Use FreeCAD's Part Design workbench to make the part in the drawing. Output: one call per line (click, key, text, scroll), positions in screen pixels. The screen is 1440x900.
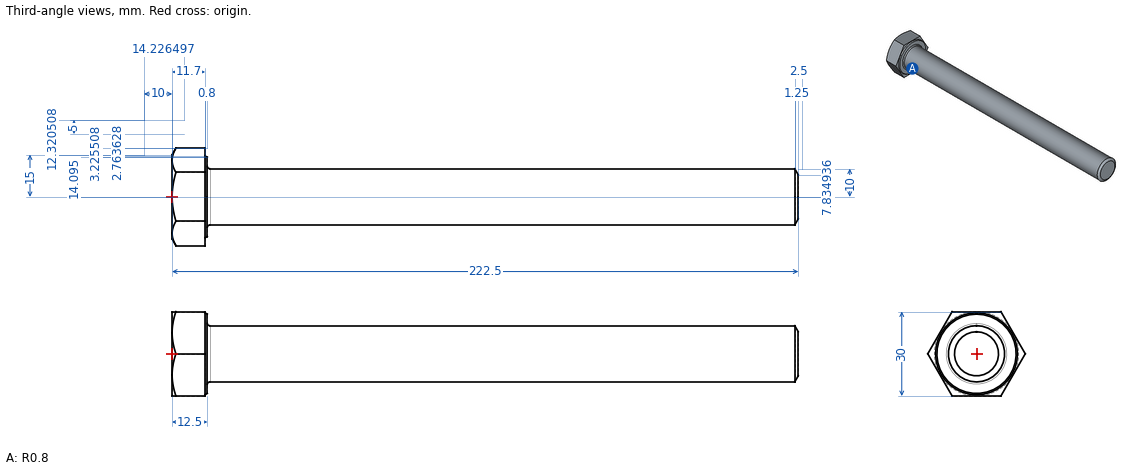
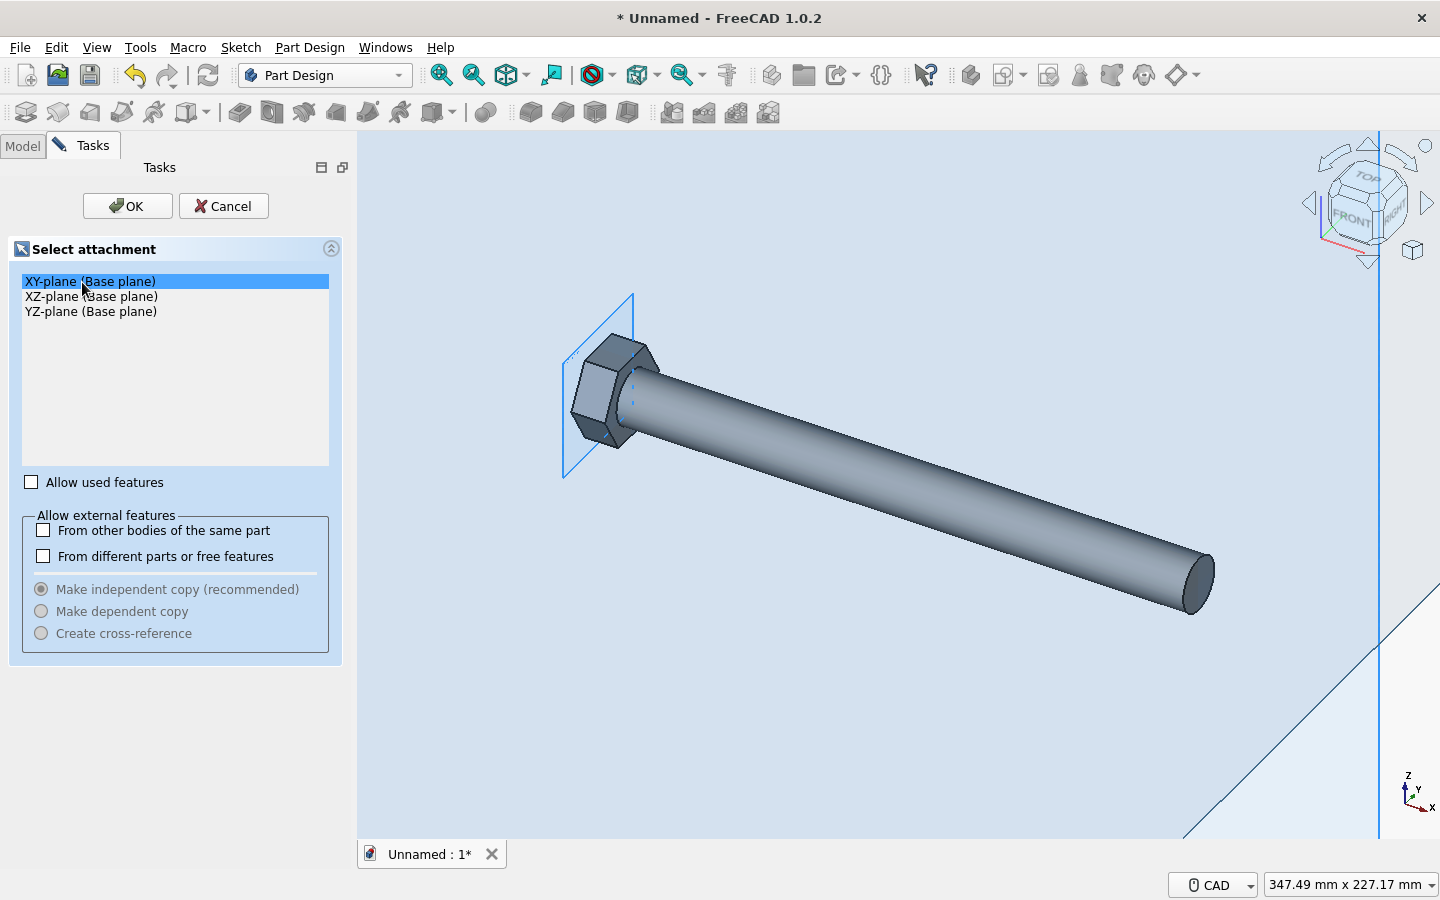
click(128, 206)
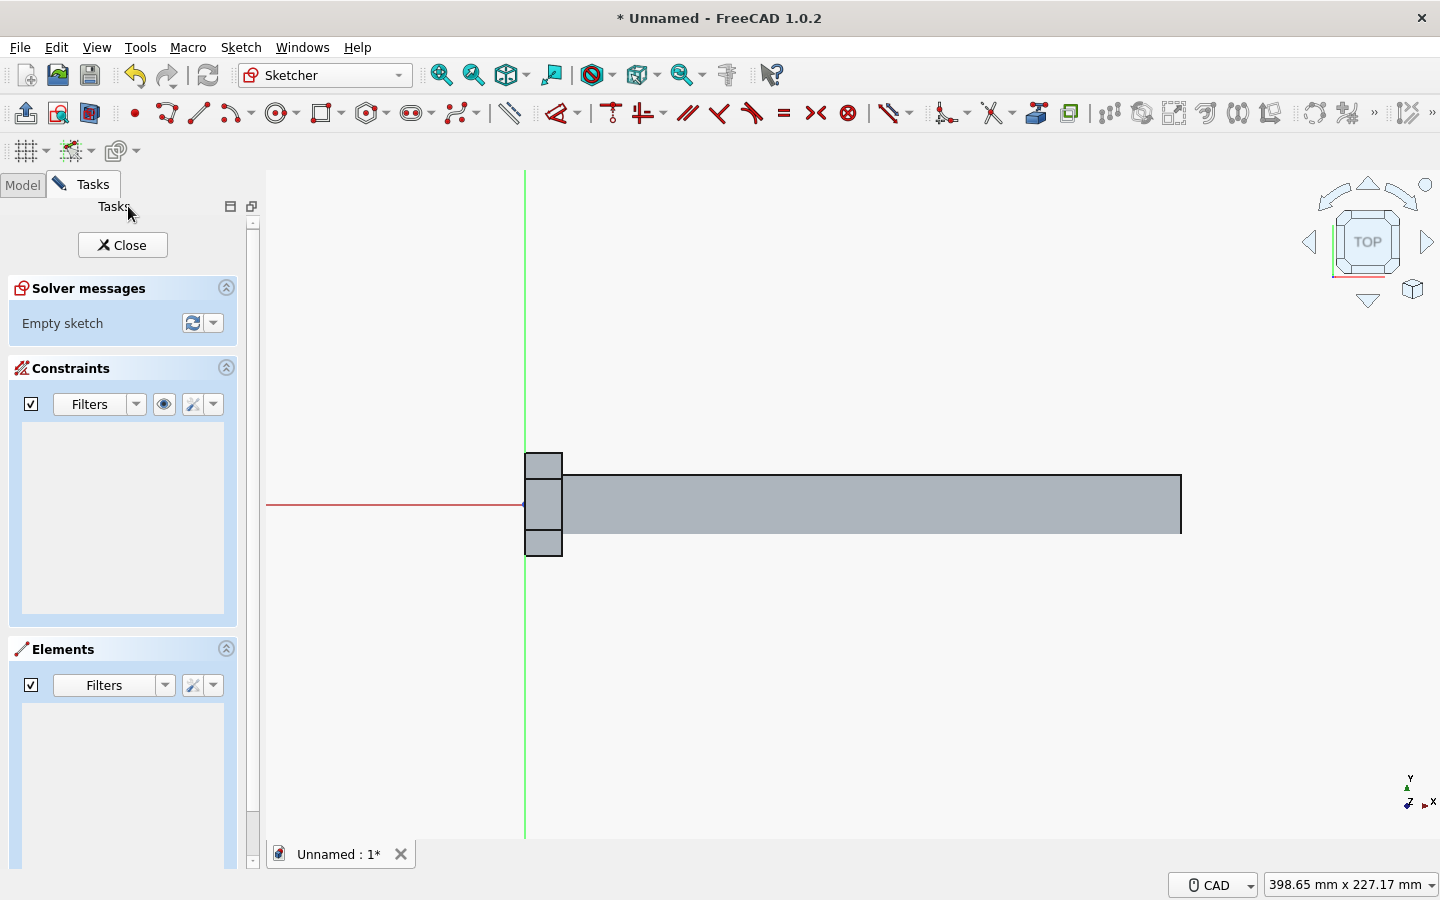
key(q)
key(s)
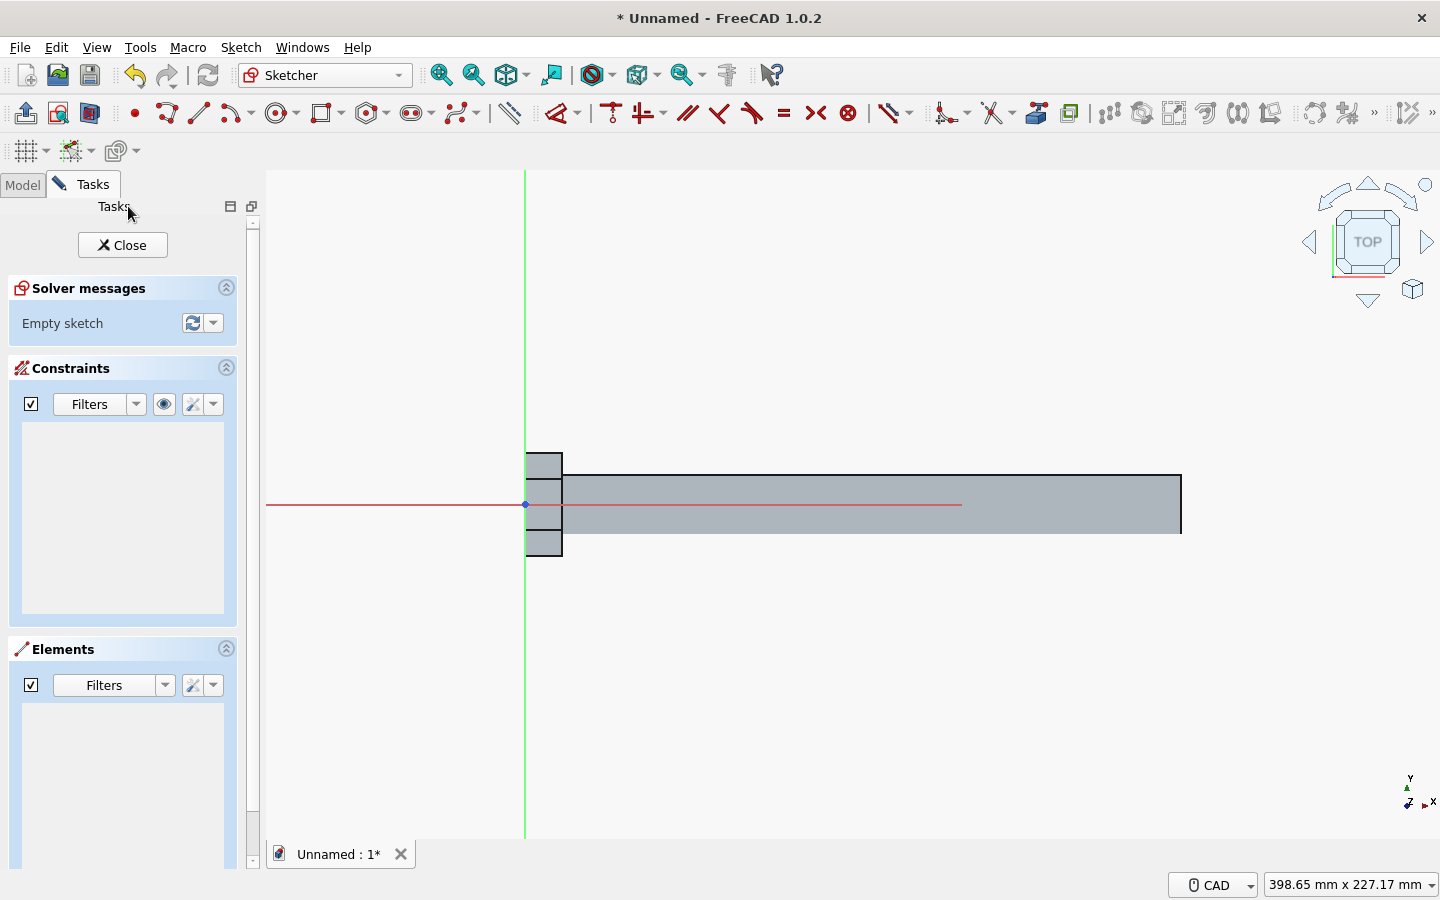
scroll(449, 454, up, 8)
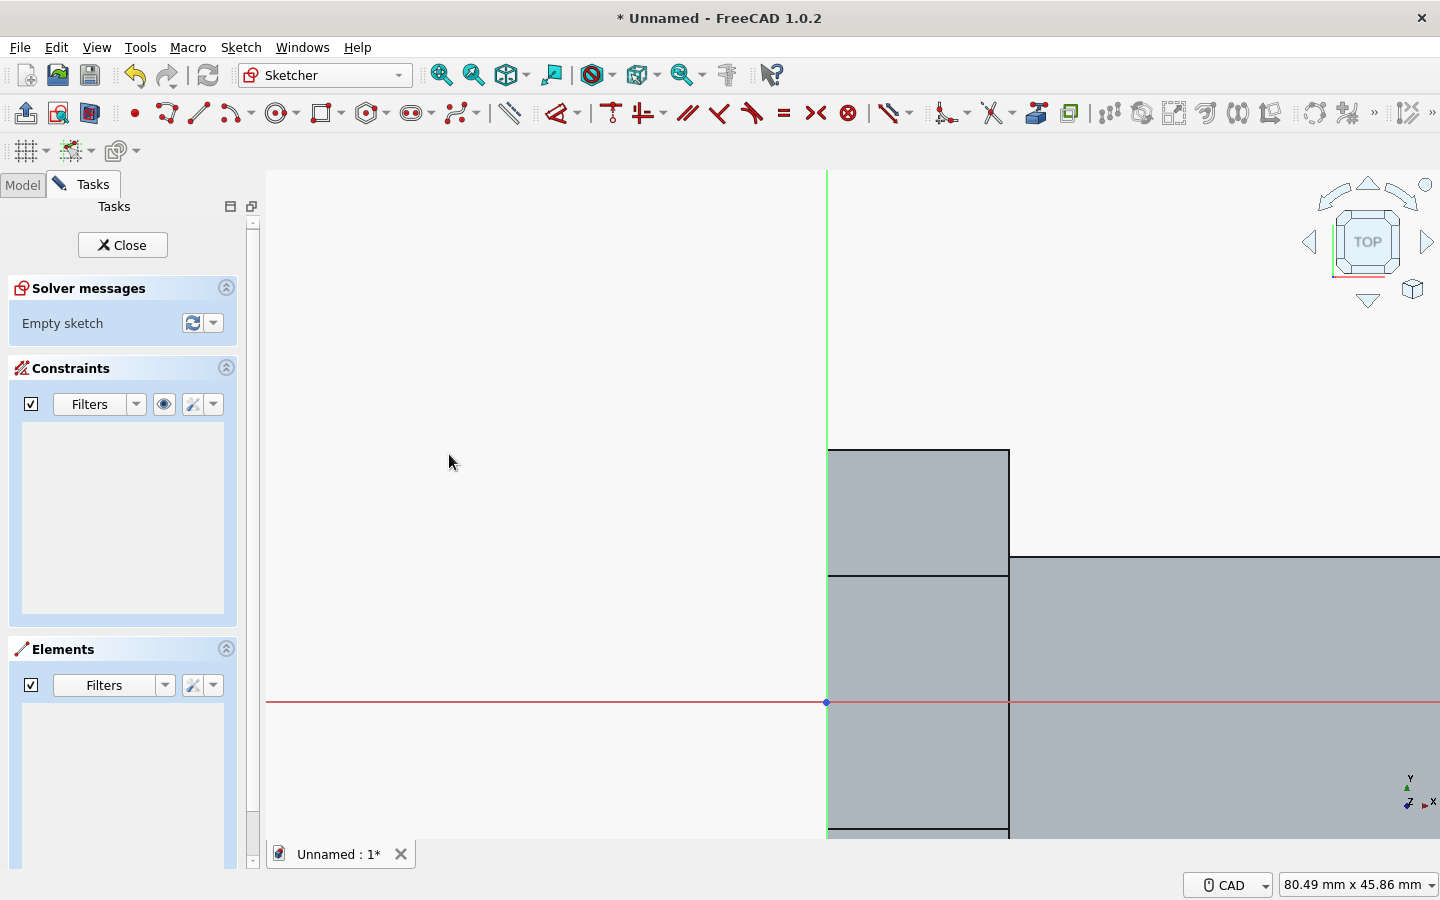
click(168, 114)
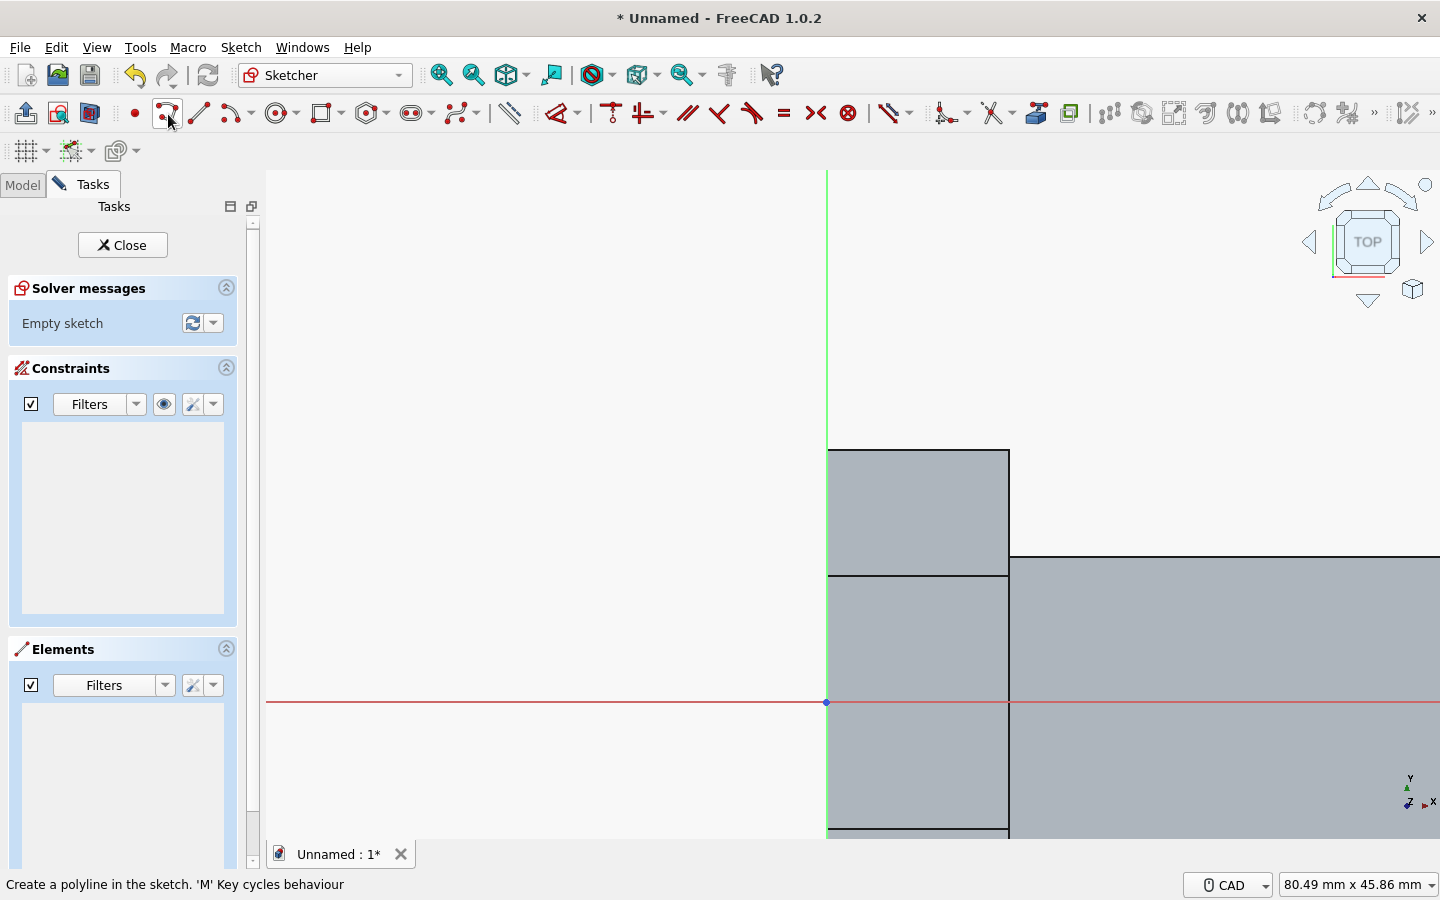
click(827, 484)
click(888, 377)
click(888, 304)
click(681, 304)
click(681, 484)
click(827, 485)
key(Escape)
key(Escape)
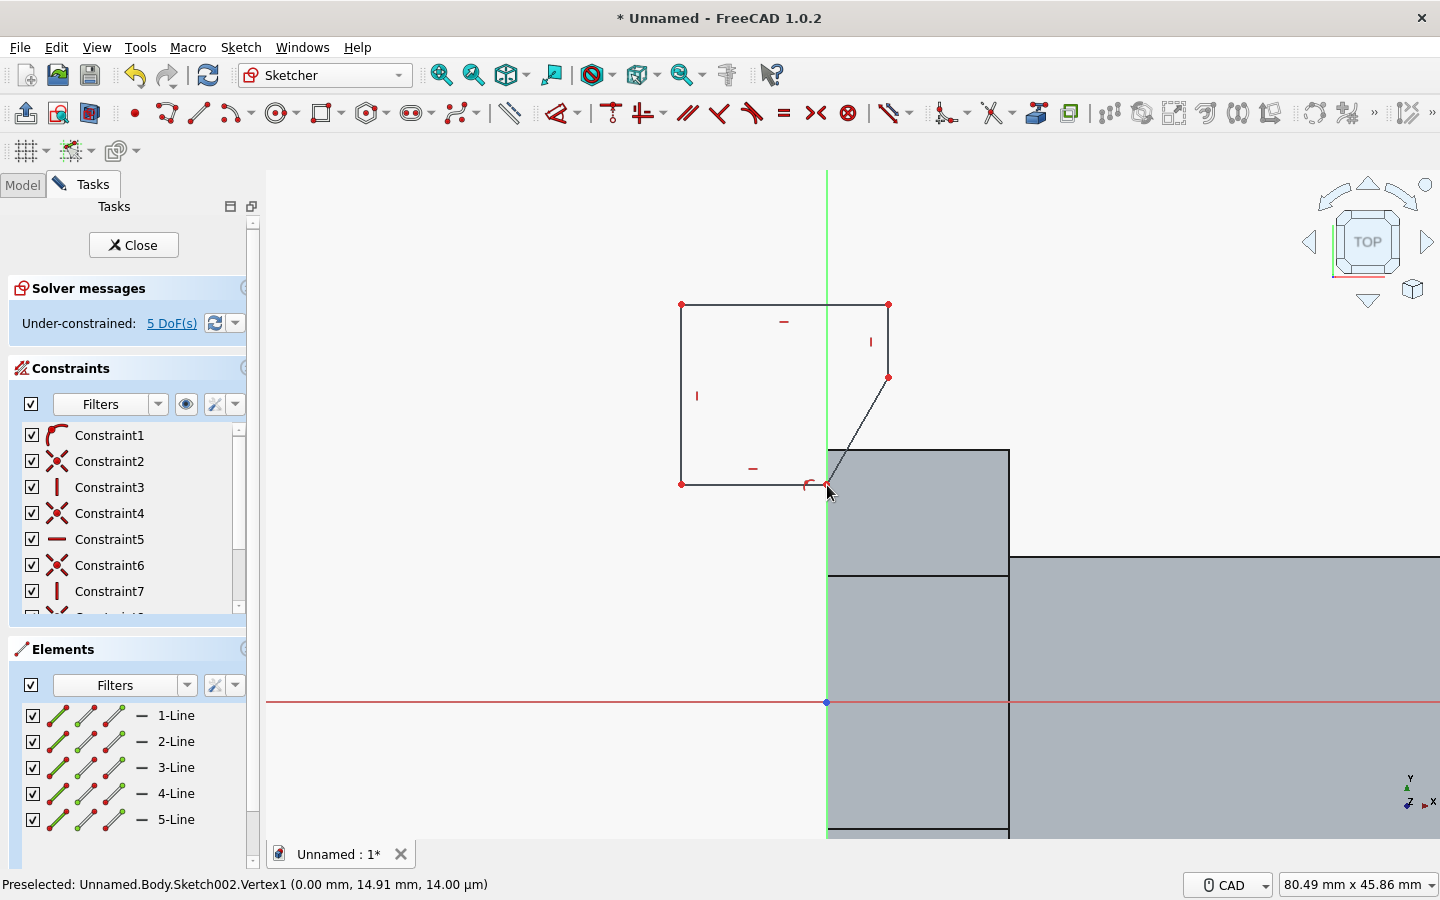
click(556, 114)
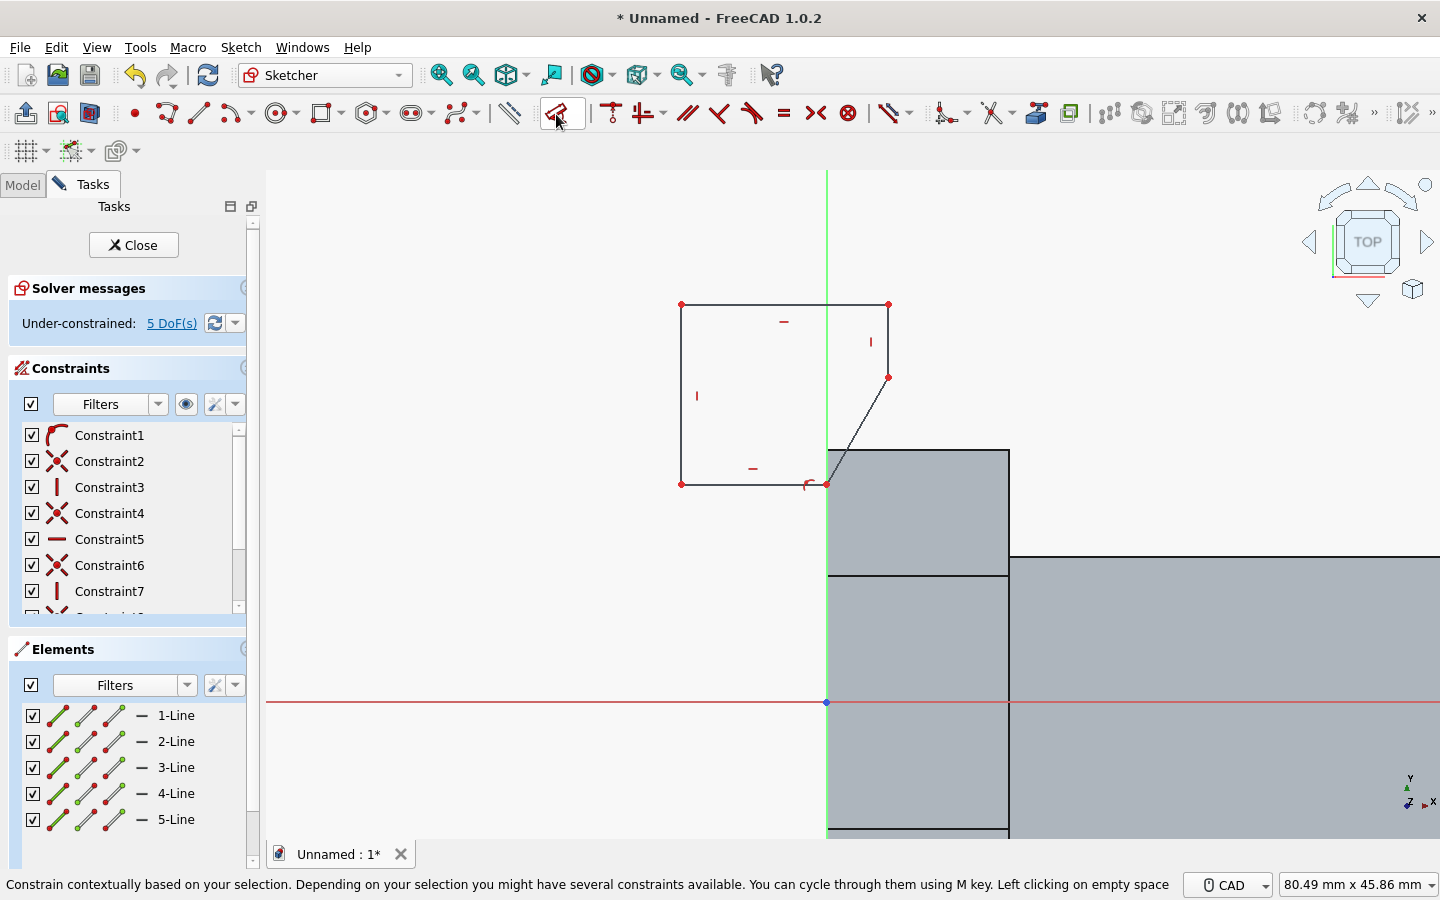
click(888, 356)
click(922, 342)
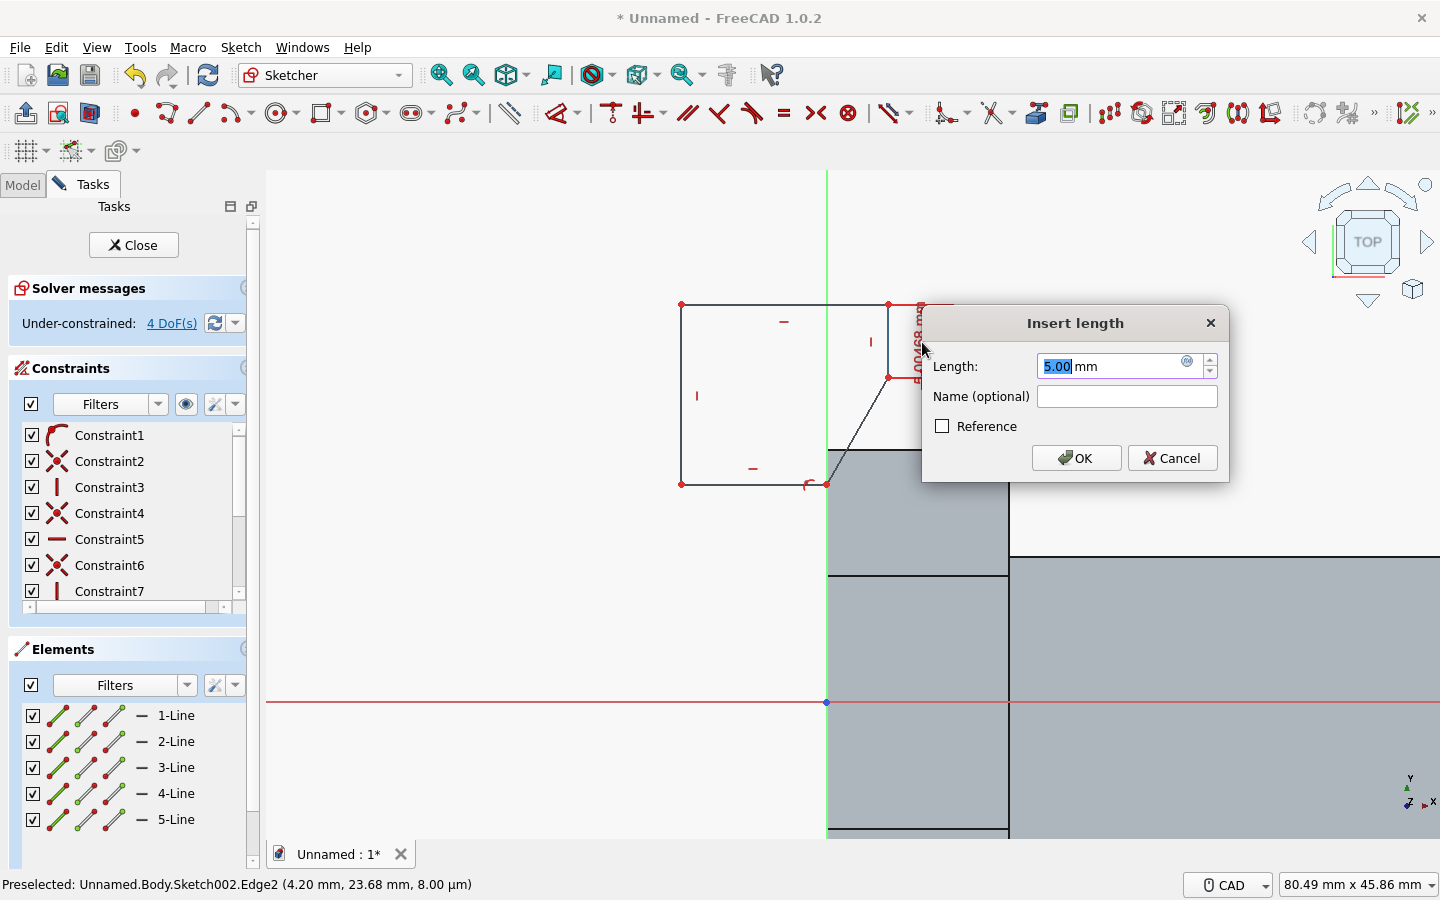
text(5)
key(Return)